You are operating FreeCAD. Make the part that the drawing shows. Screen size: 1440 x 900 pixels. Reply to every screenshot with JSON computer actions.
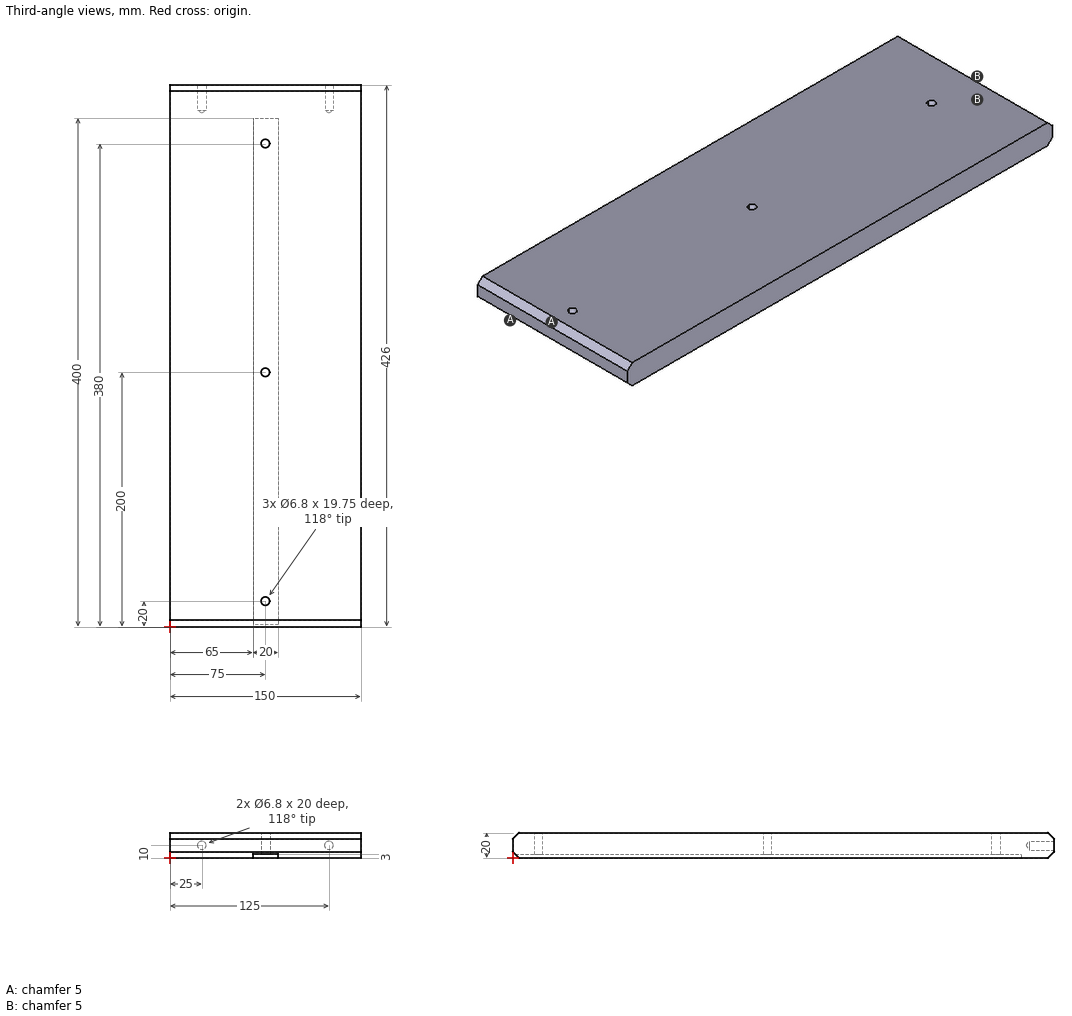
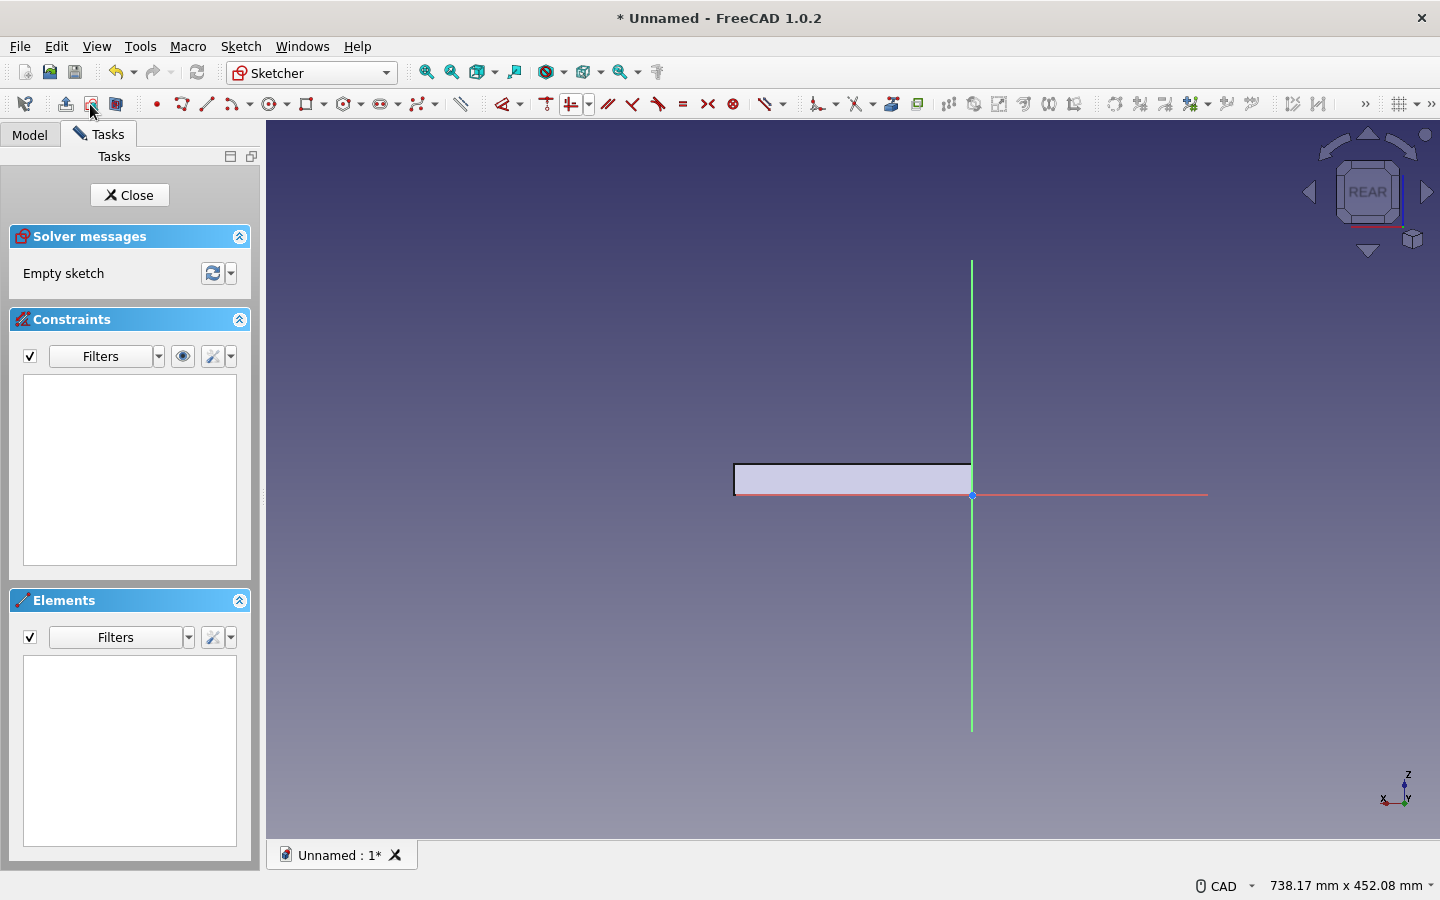
{"action": "scroll", "coordinate": [907, 487], "scroll_direction": "up", "scroll_amount": 6}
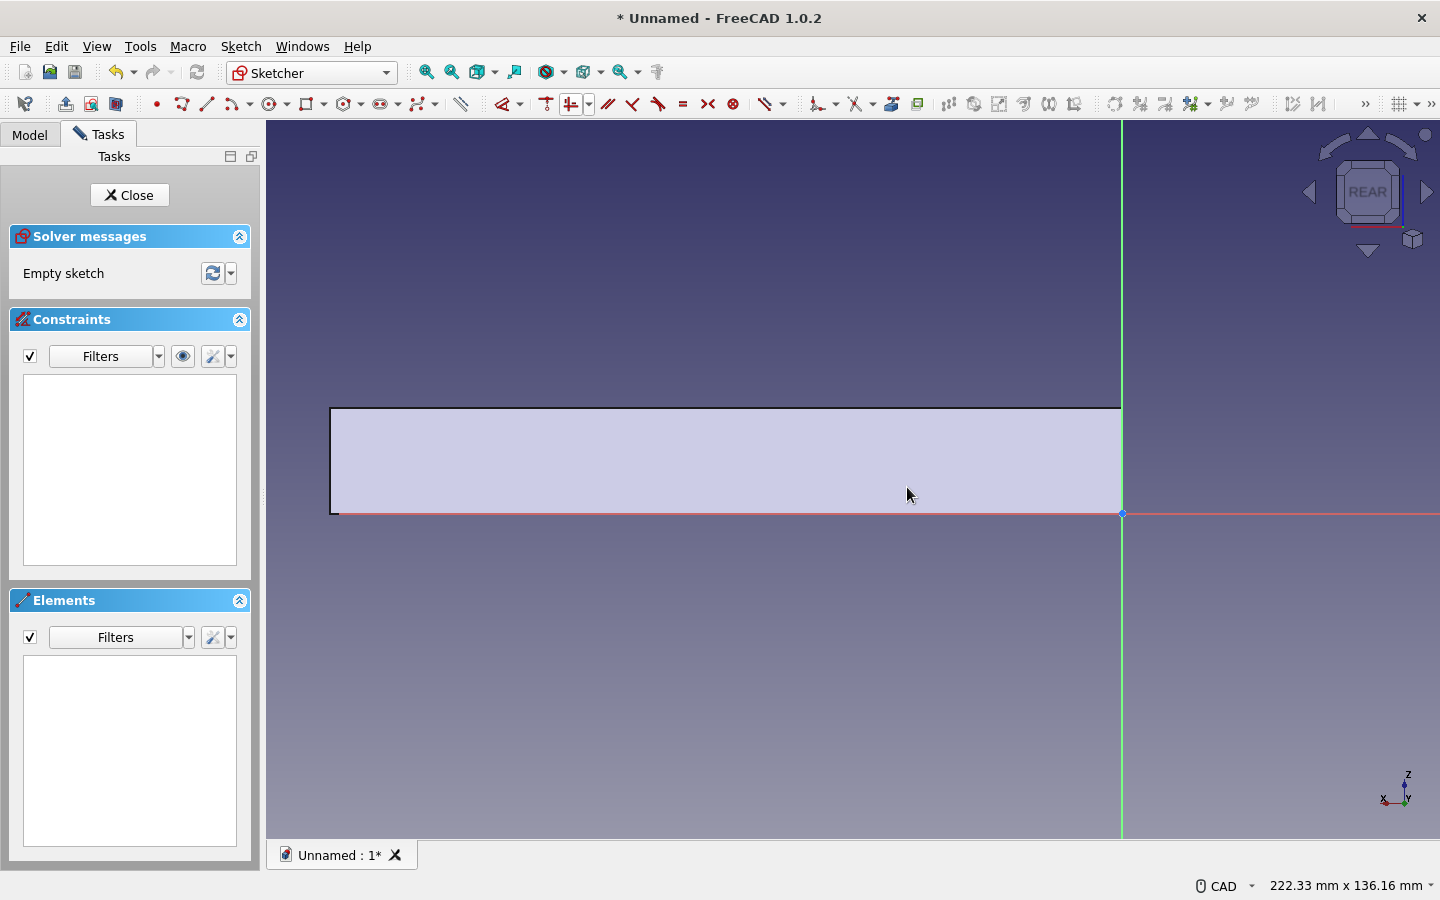
{"action": "key", "text": "g c"}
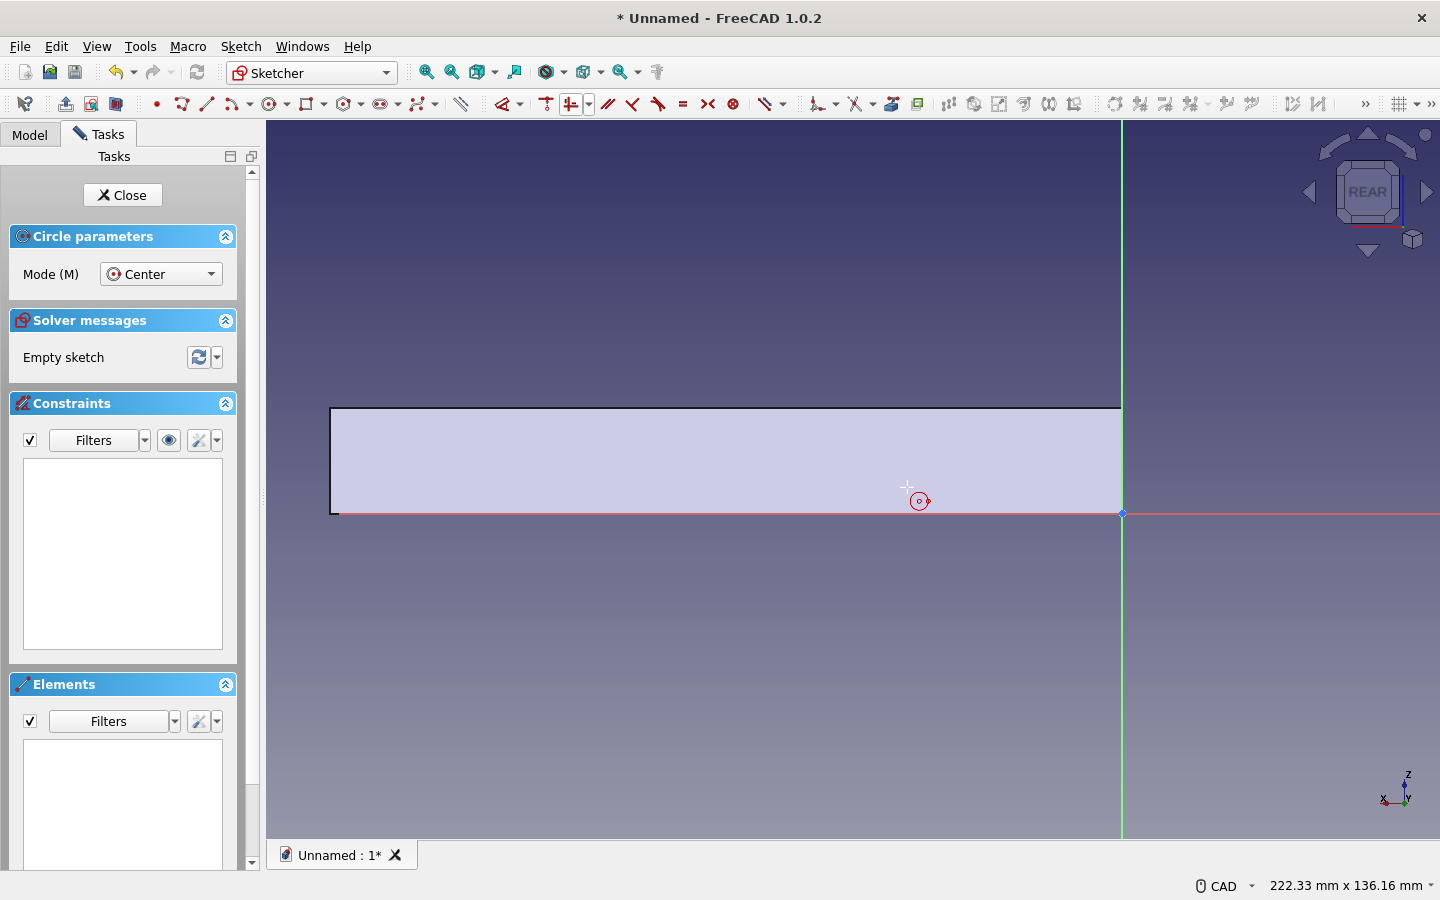
{"action": "scroll", "coordinate": [990, 461], "scroll_direction": "up", "scroll_amount": 2}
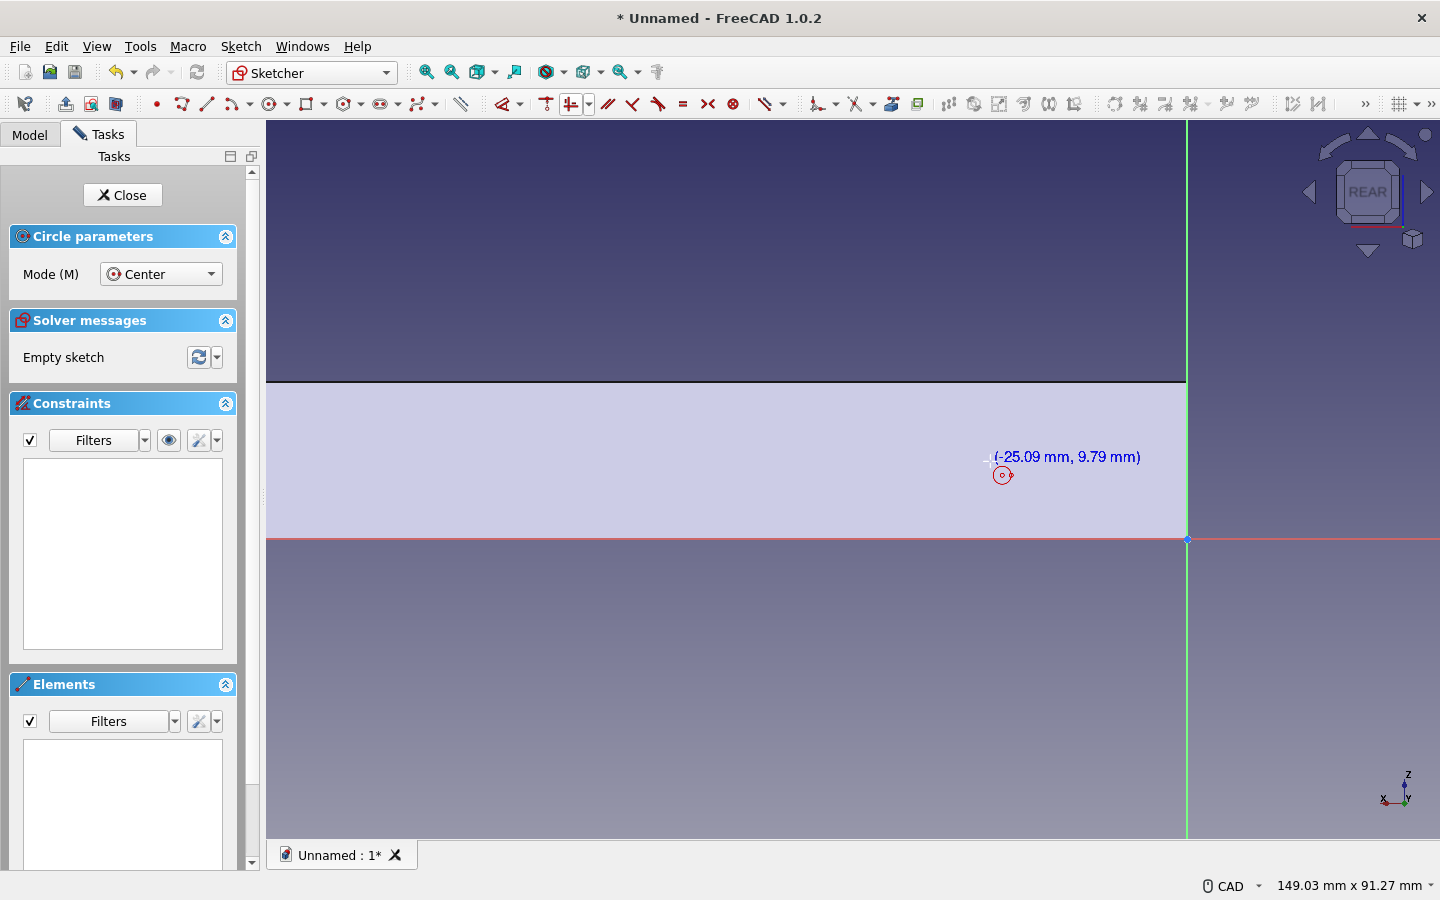
{"action": "left_click", "coordinate": [990, 461]}
{"action": "left_click", "coordinate": [1009, 442]}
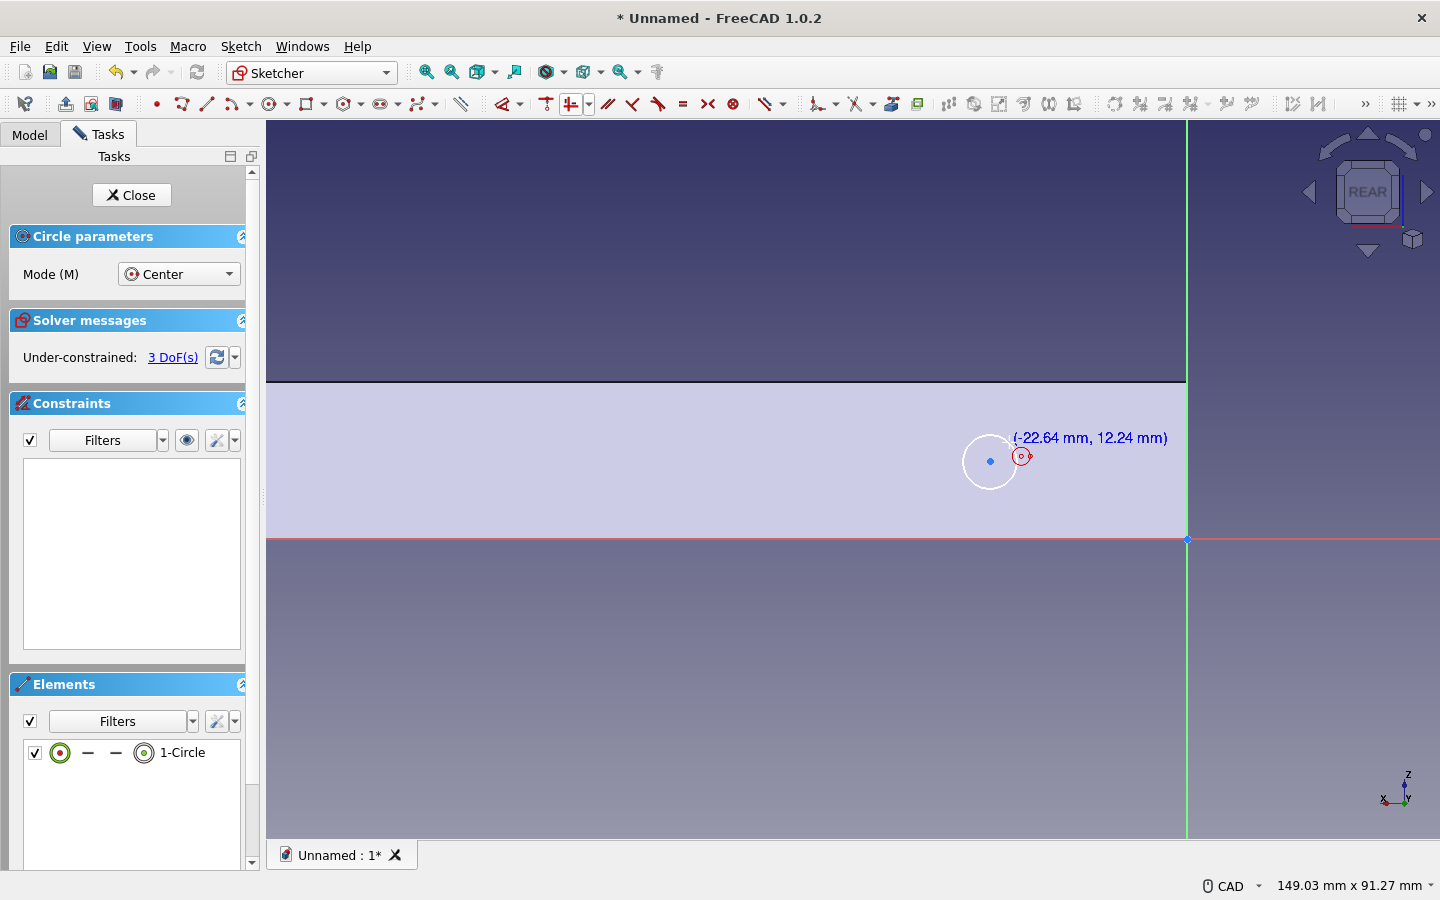
{"action": "scroll", "coordinate": [994, 465], "scroll_direction": "down", "scroll_amount": 2}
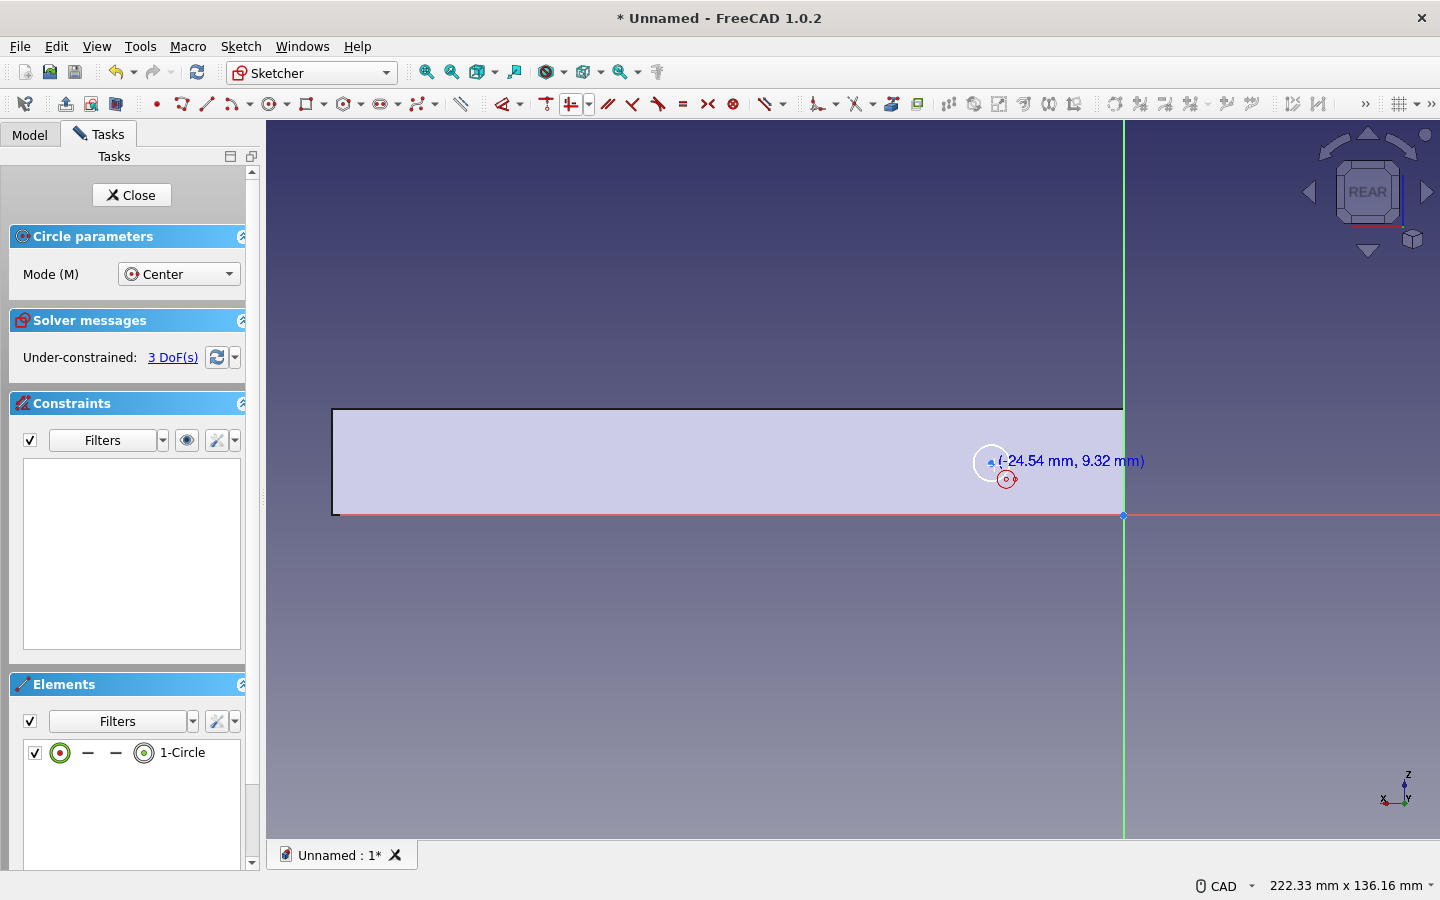
{"action": "scroll", "coordinate": [464, 462], "scroll_direction": "up", "scroll_amount": 2}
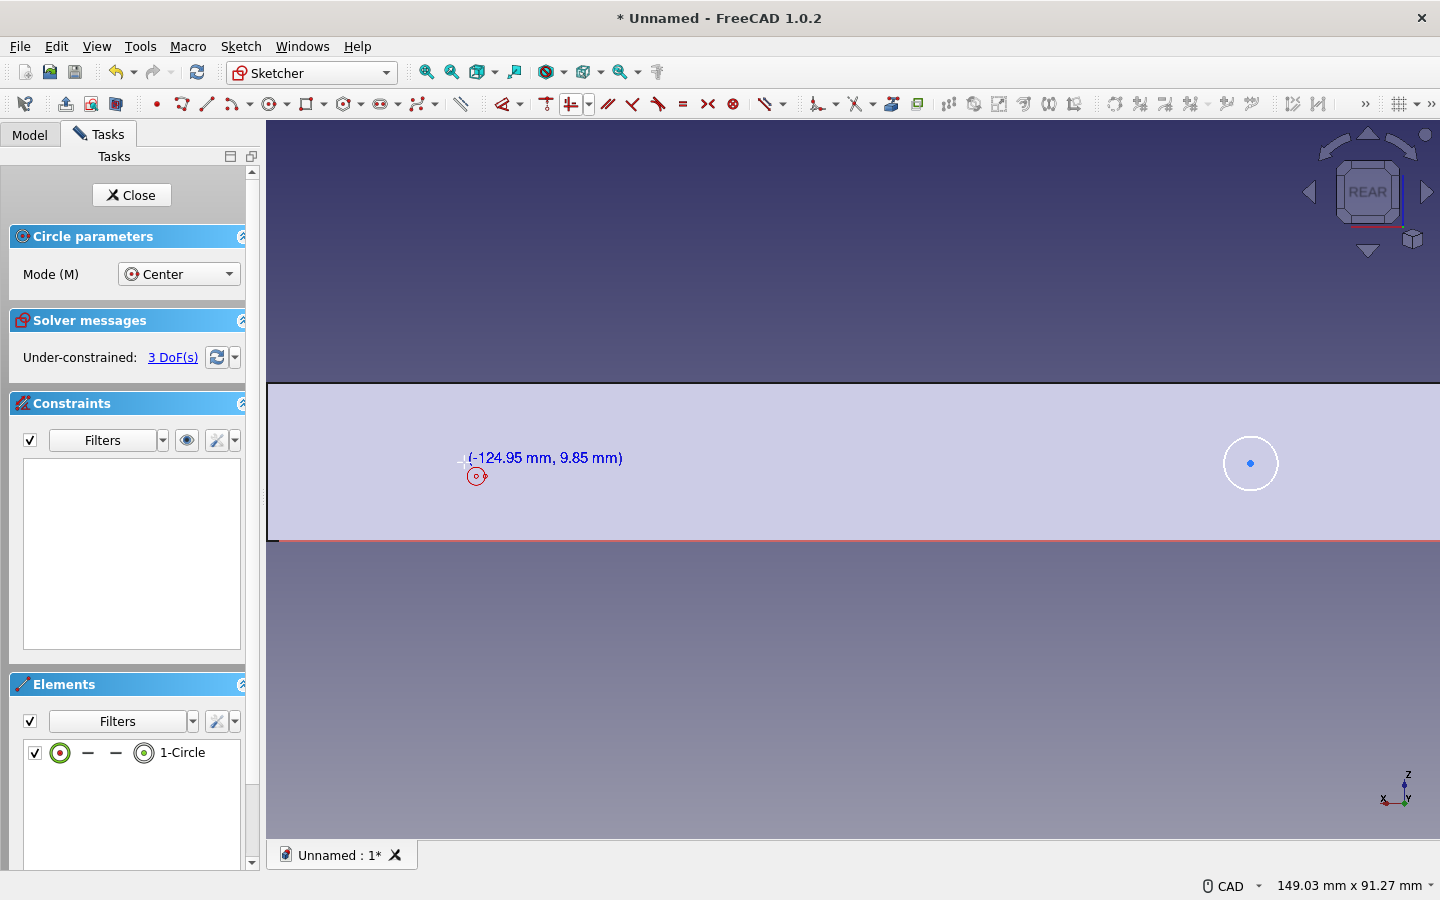
{"action": "left_click", "coordinate": [464, 462]}
{"action": "left_click", "coordinate": [482, 443]}
{"action": "key", "text": "Escape"}